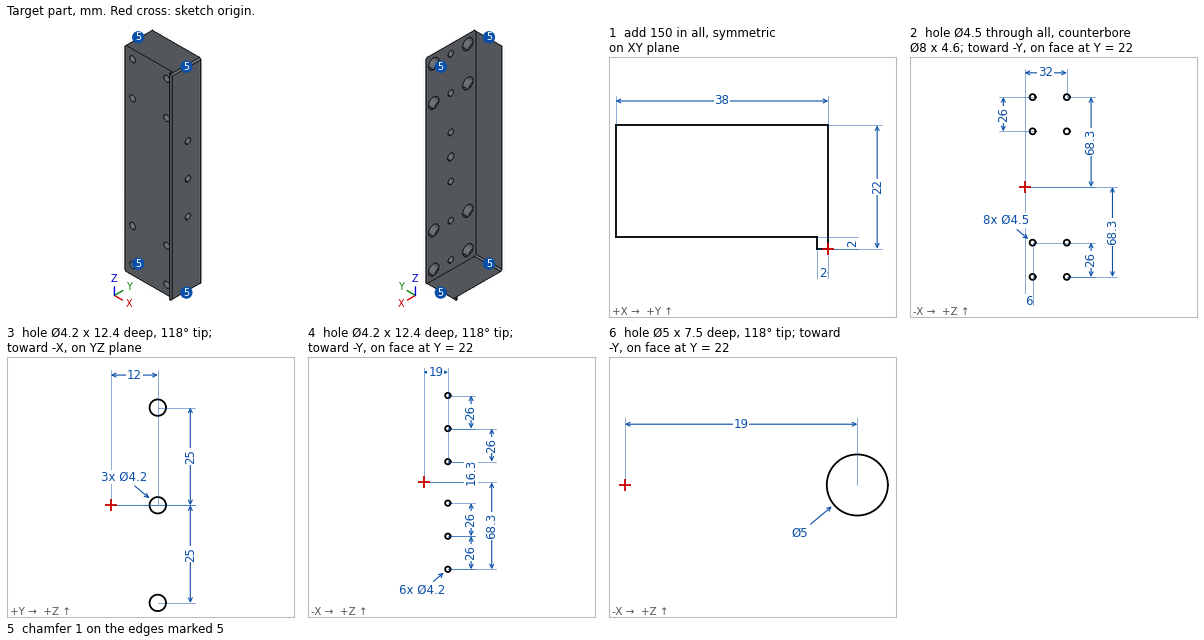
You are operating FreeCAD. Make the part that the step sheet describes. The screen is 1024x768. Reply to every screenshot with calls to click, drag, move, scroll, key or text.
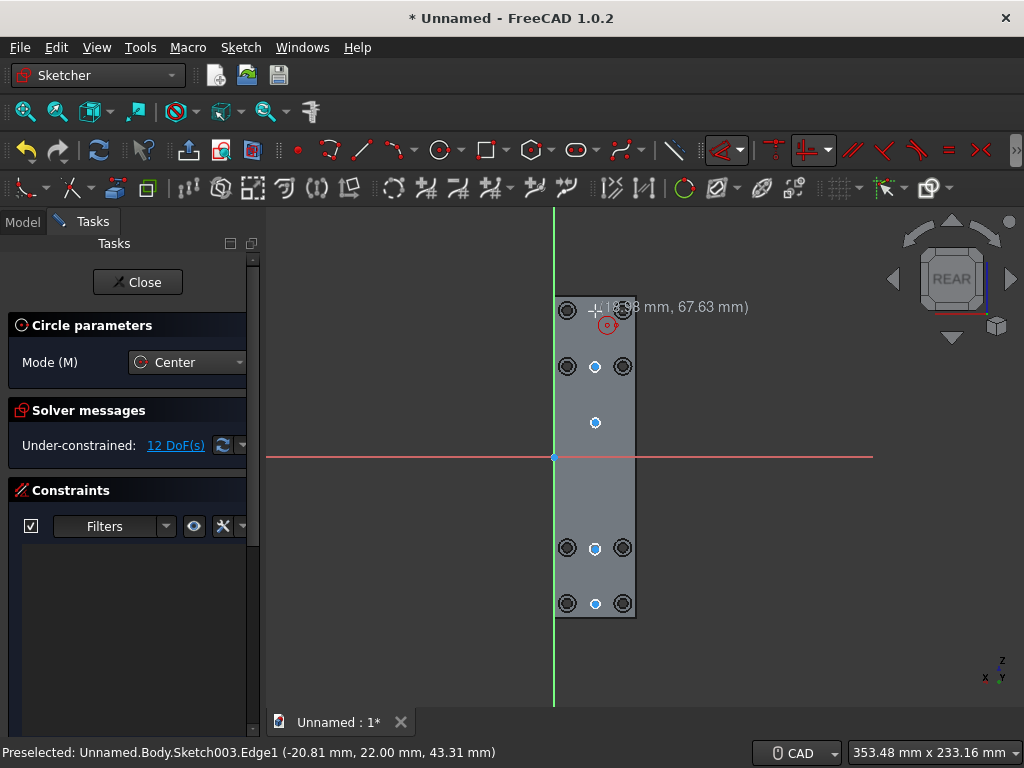
click(595, 311)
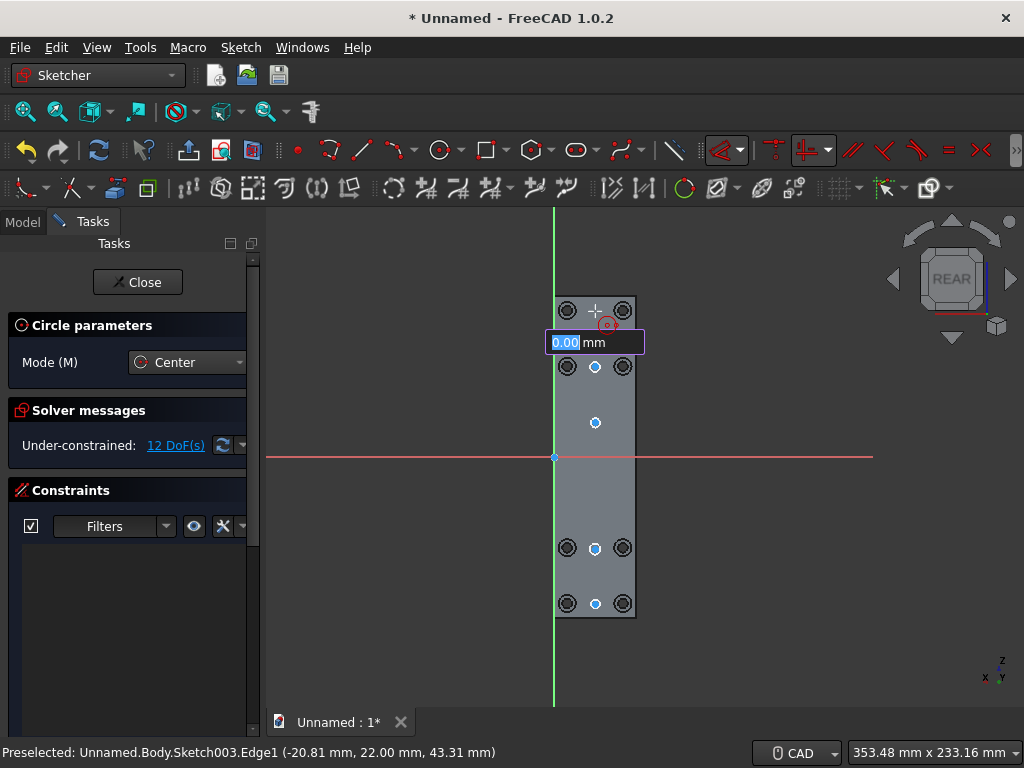
scroll(598, 307, up, 7)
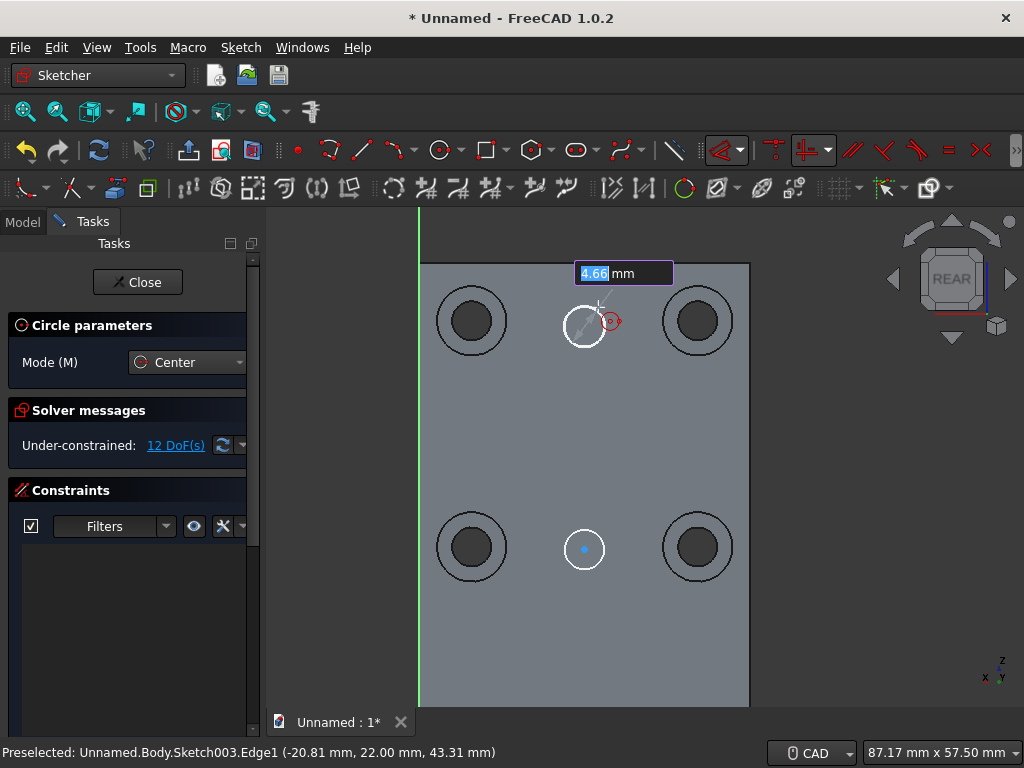
click(598, 308)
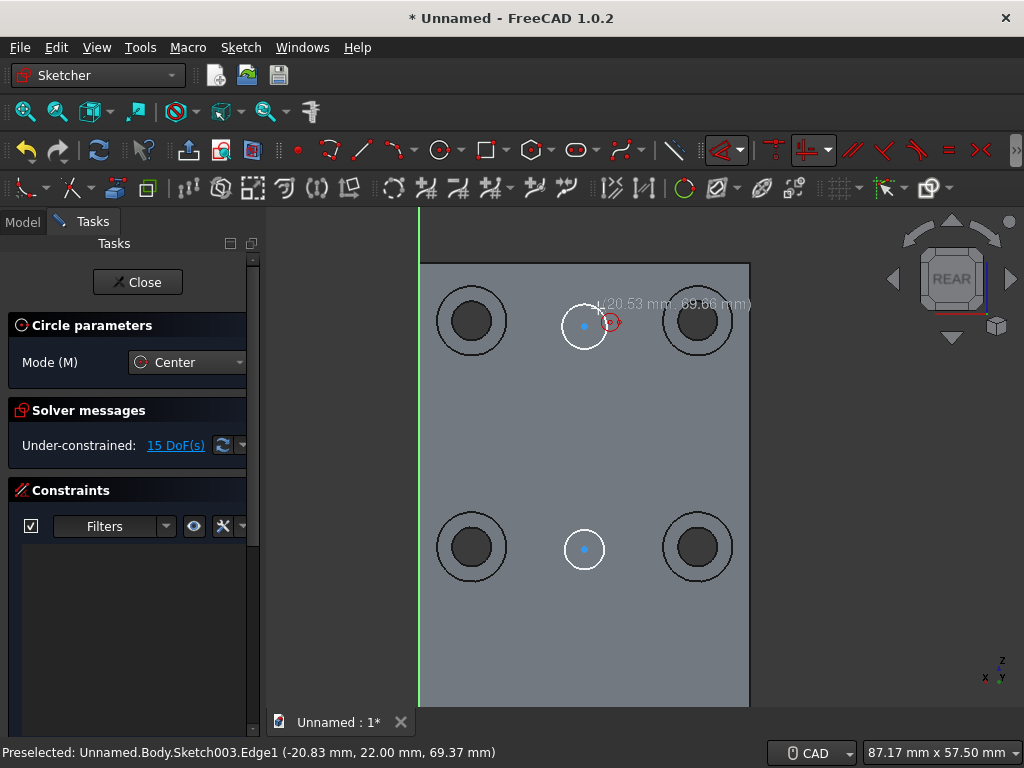
scroll(598, 307, down, 7)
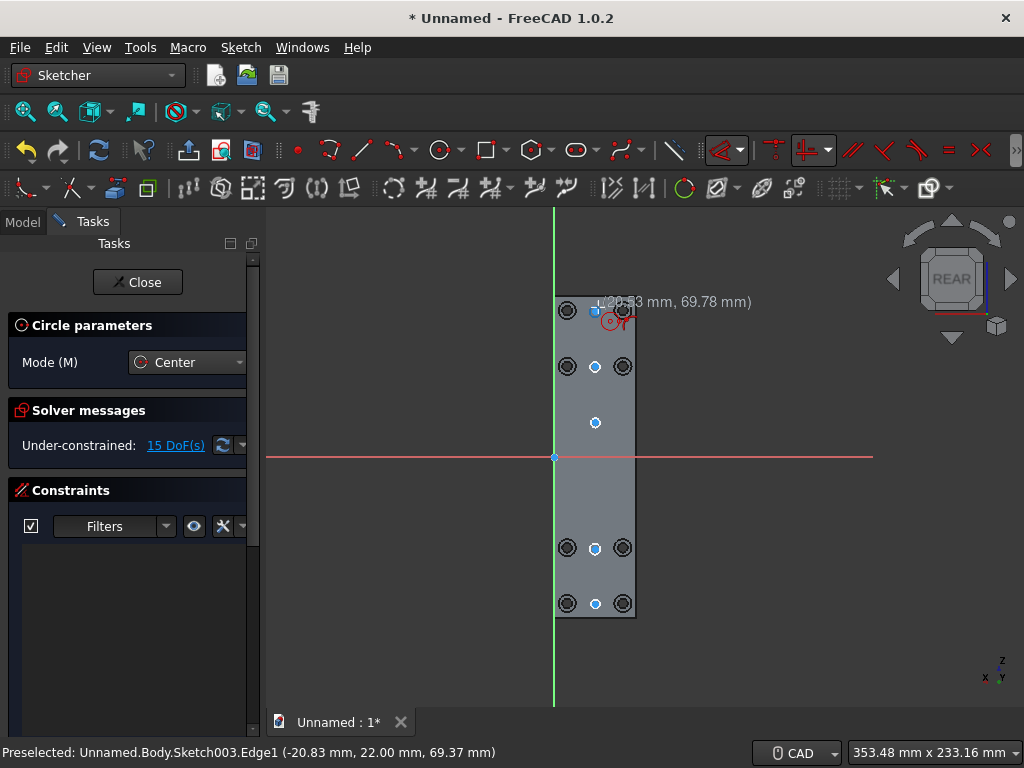
scroll(595, 492, up, 9)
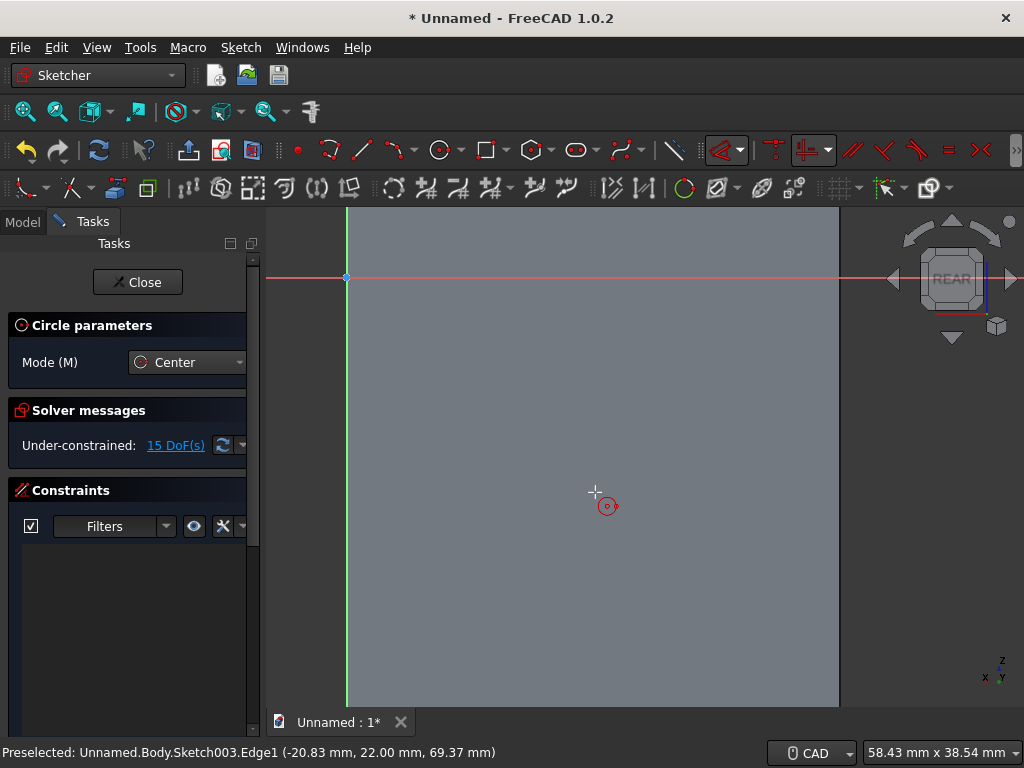
scroll(595, 493, down, 9)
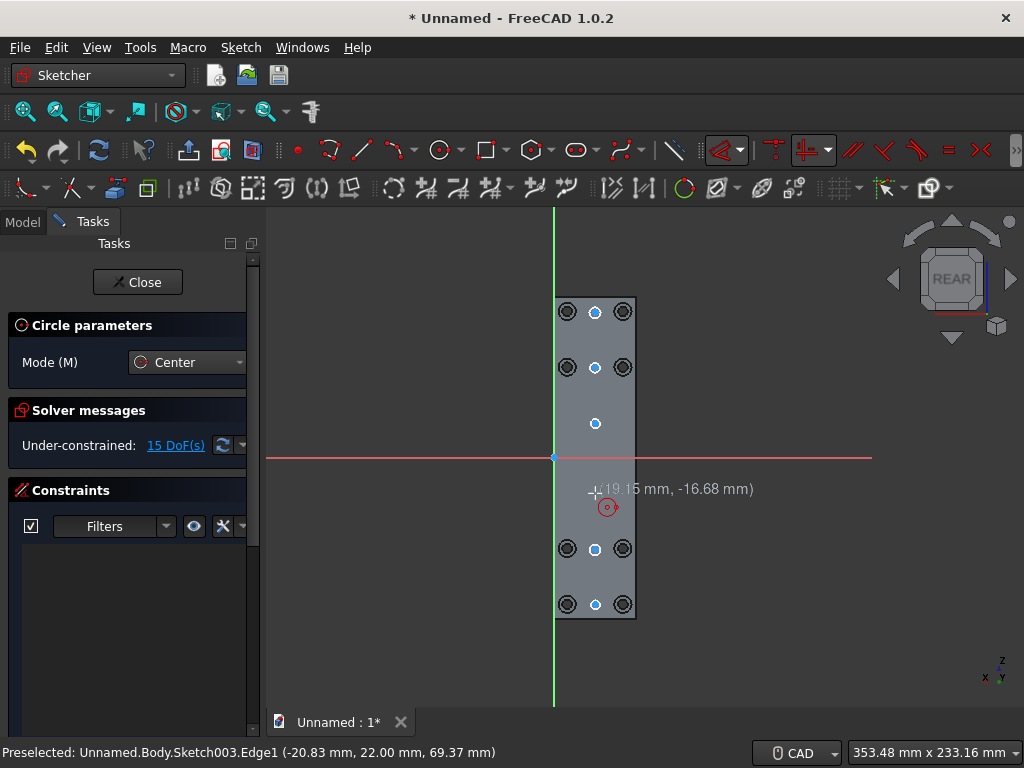
click(595, 493)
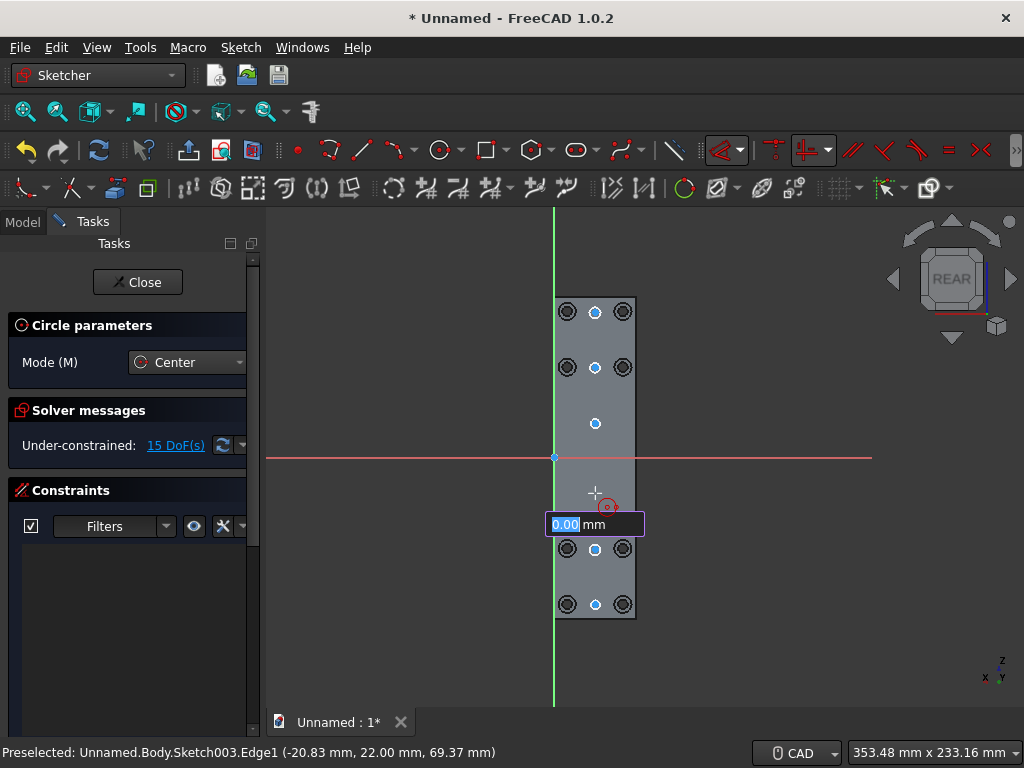
scroll(598, 490, up, 7)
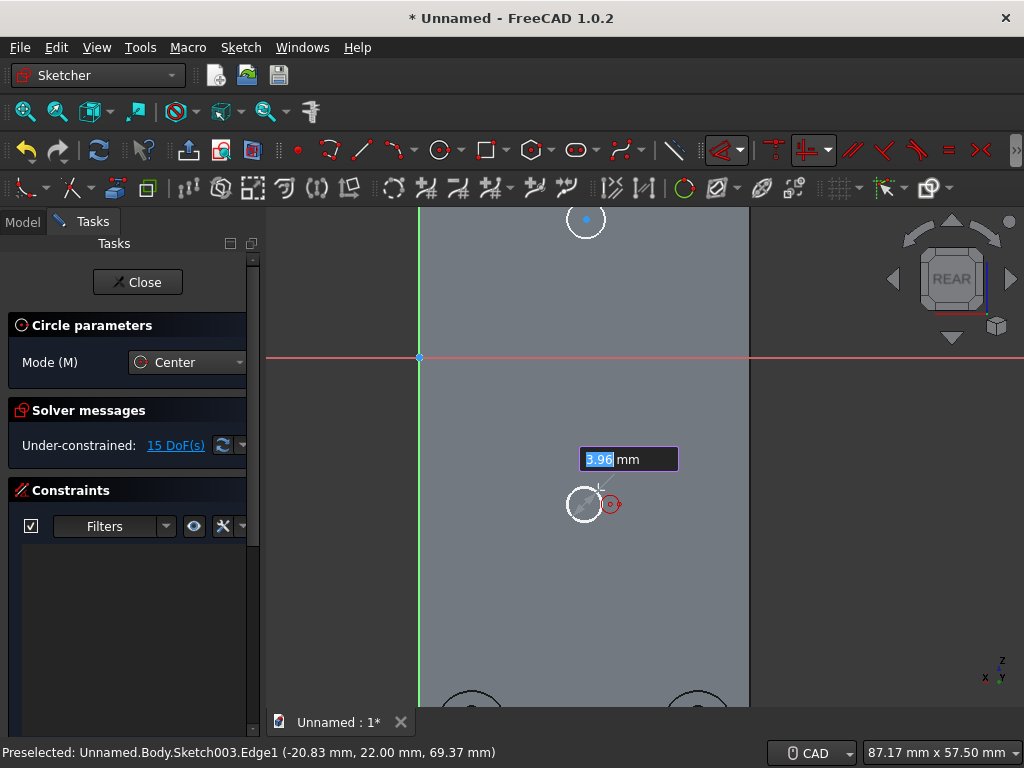
click(598, 487)
key(Escape)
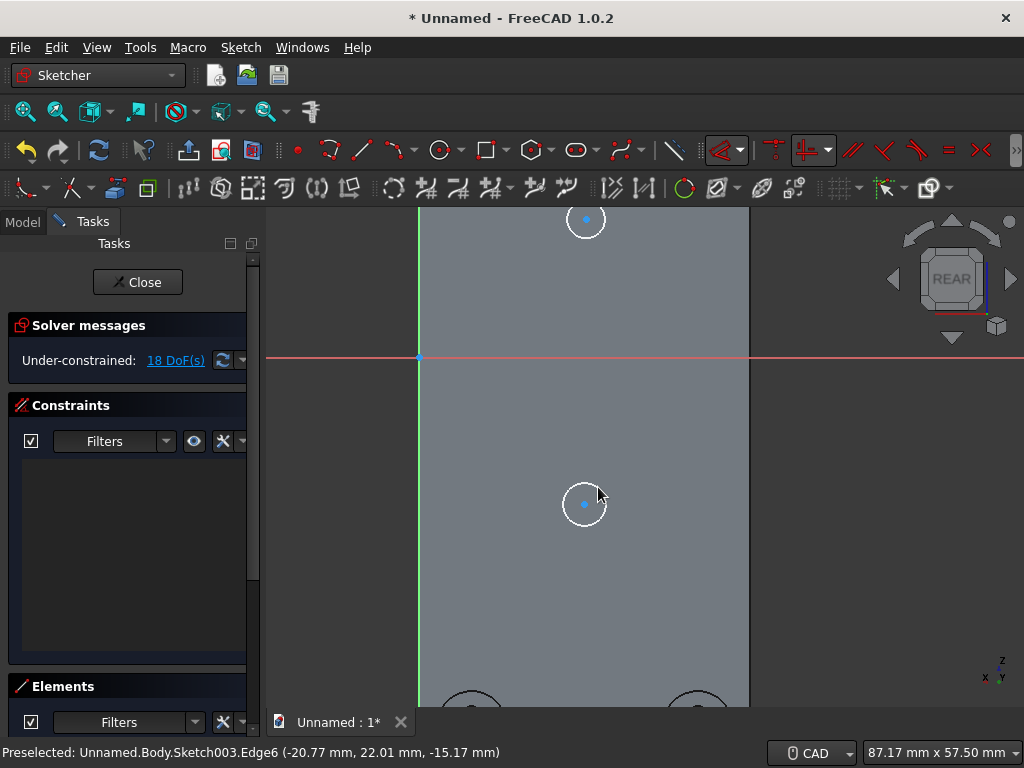
click(586, 238)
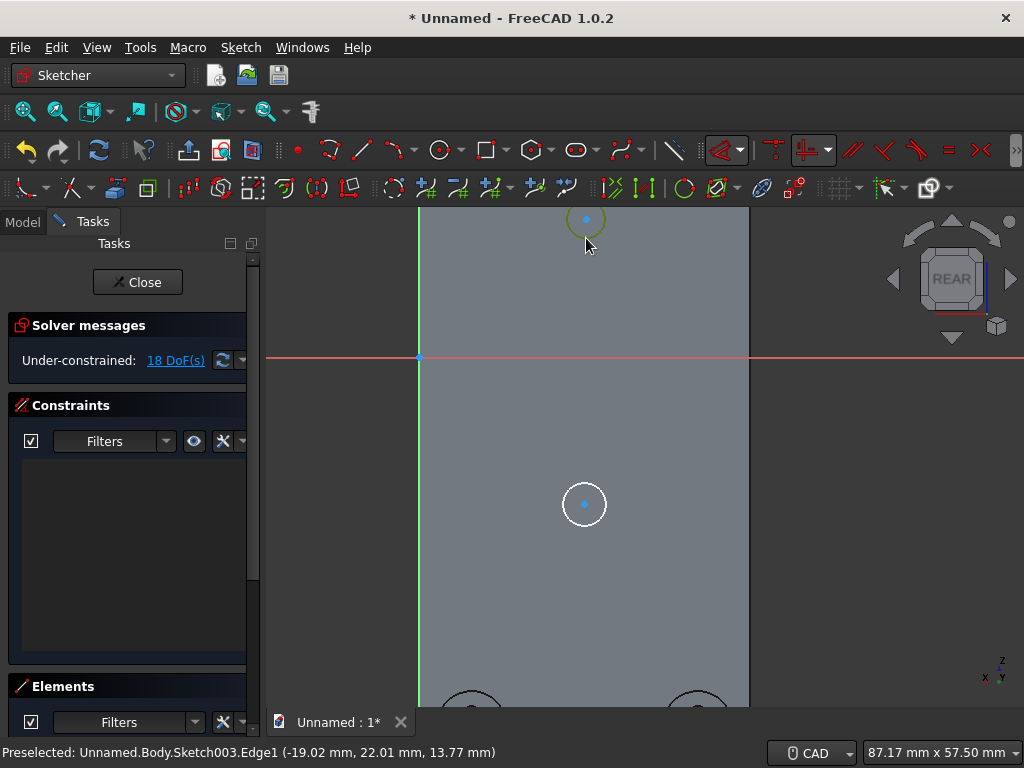
scroll(598, 489, down, 7)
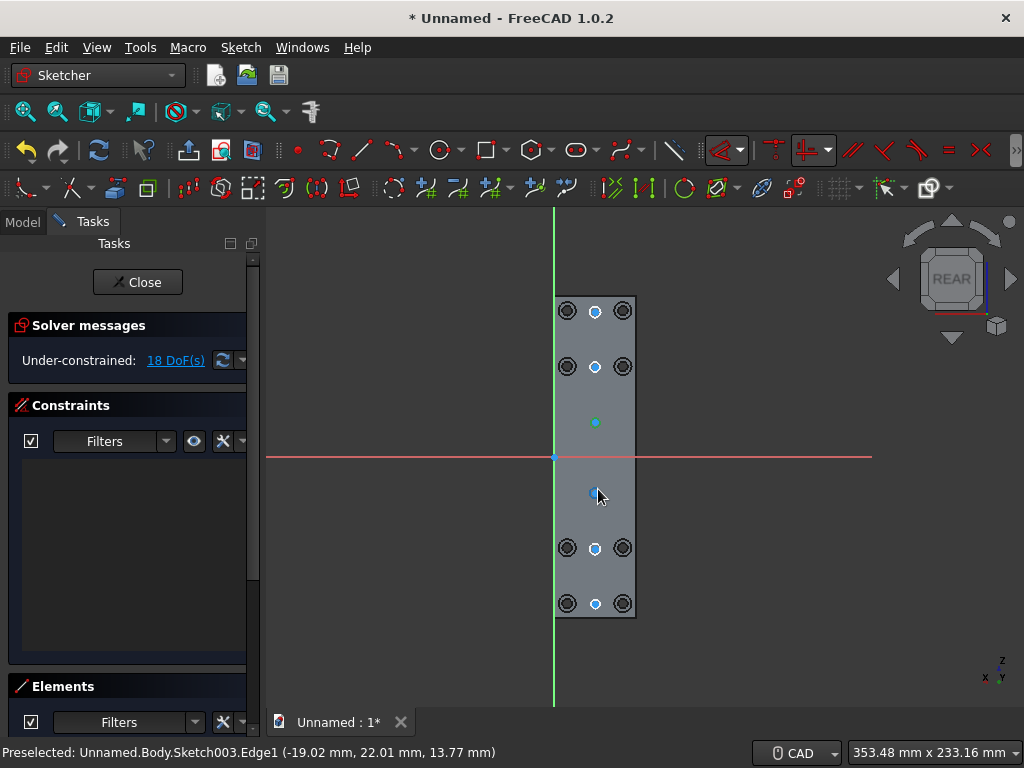
scroll(599, 601, up, 6)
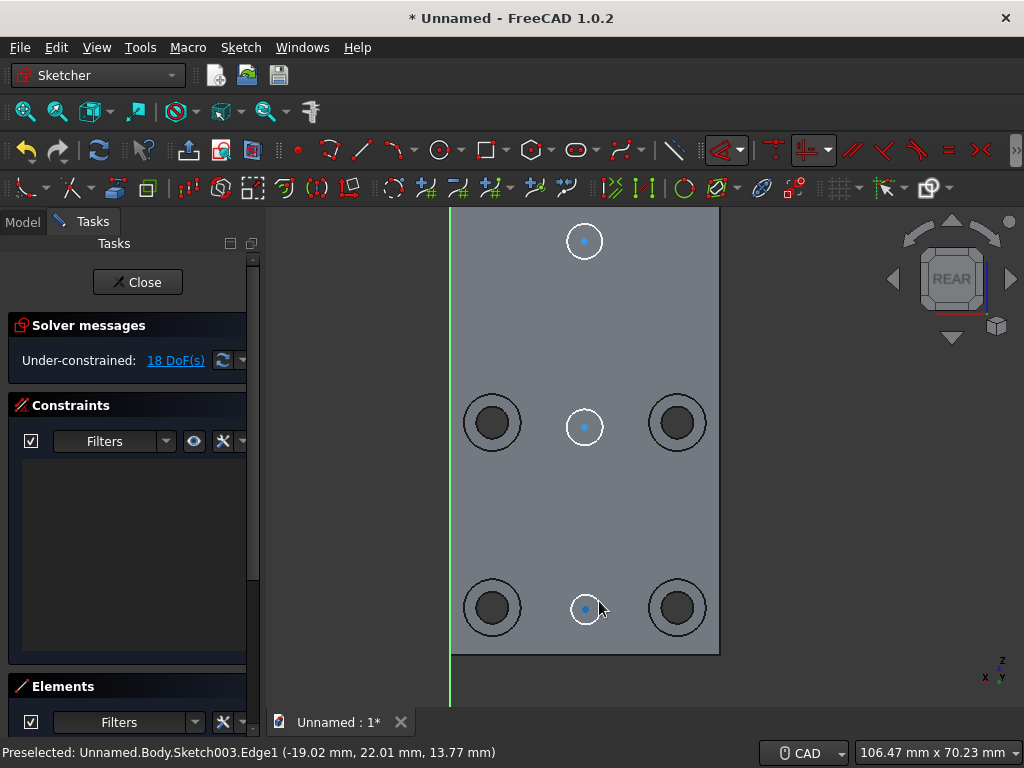
click(596, 599)